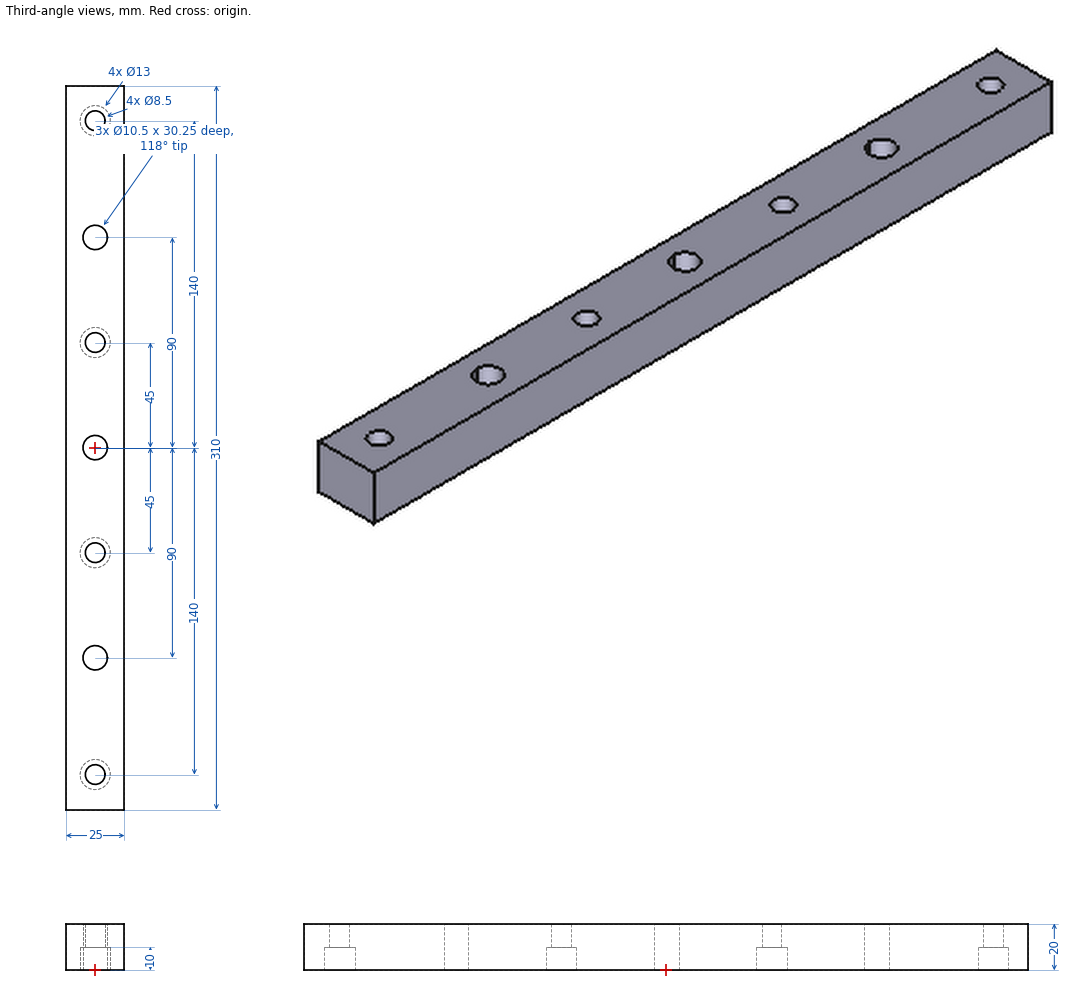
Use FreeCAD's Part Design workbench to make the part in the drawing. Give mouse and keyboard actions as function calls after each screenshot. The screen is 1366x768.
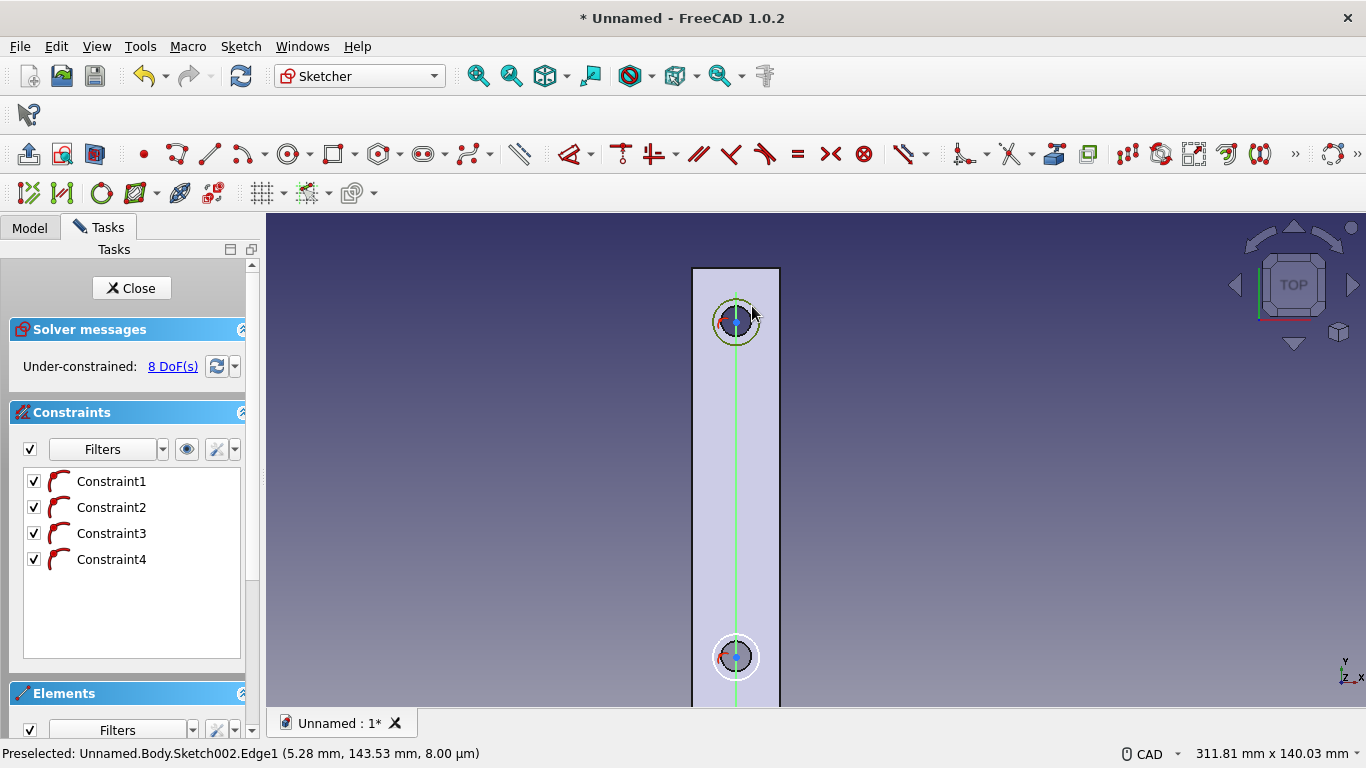
click(752, 641)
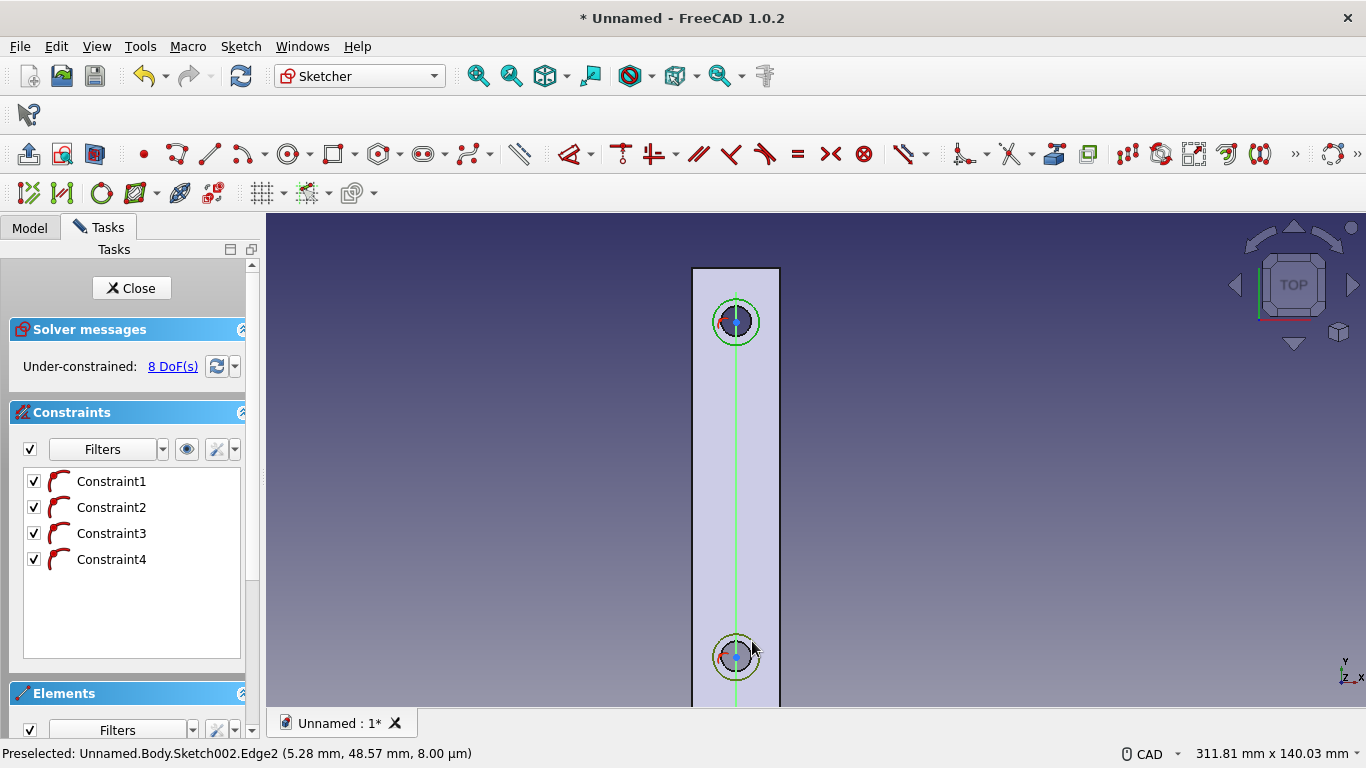
scroll(752, 307, down, 6)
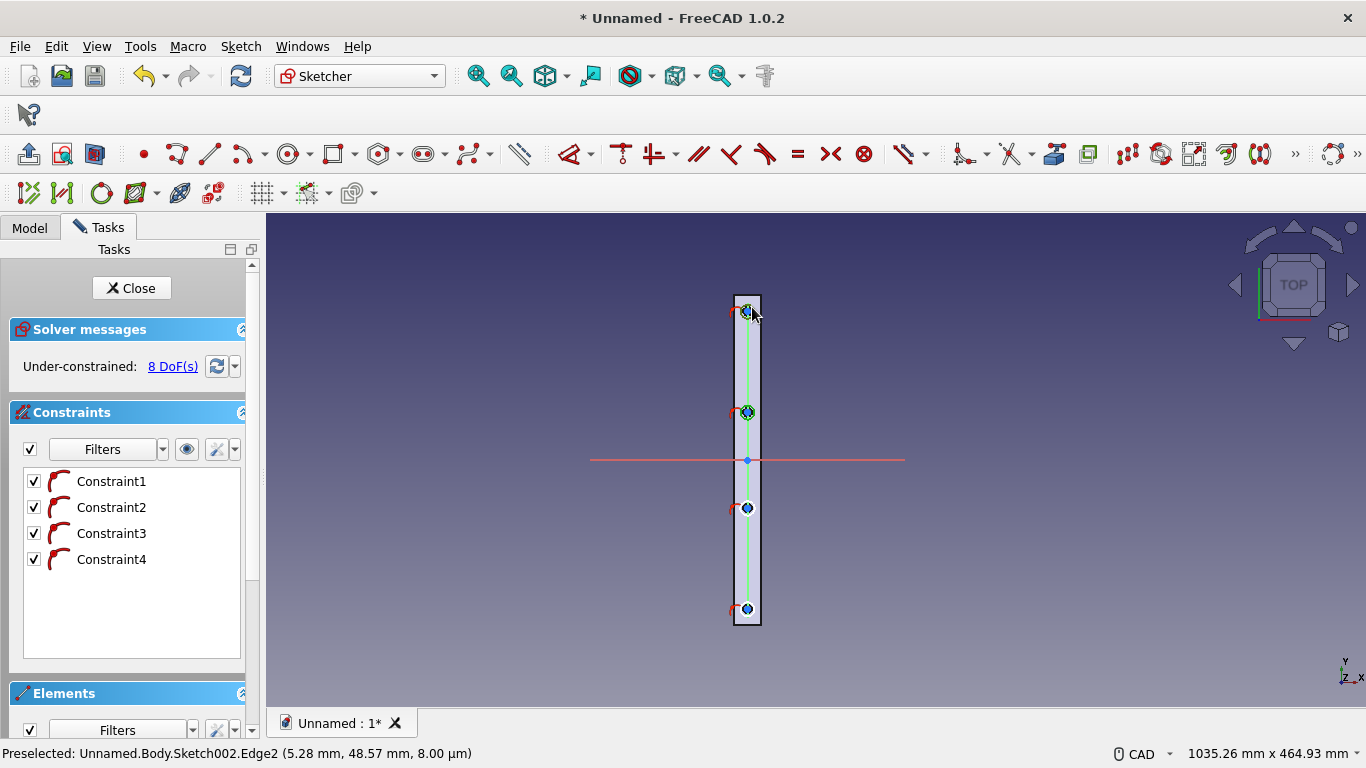
scroll(753, 503, up, 6)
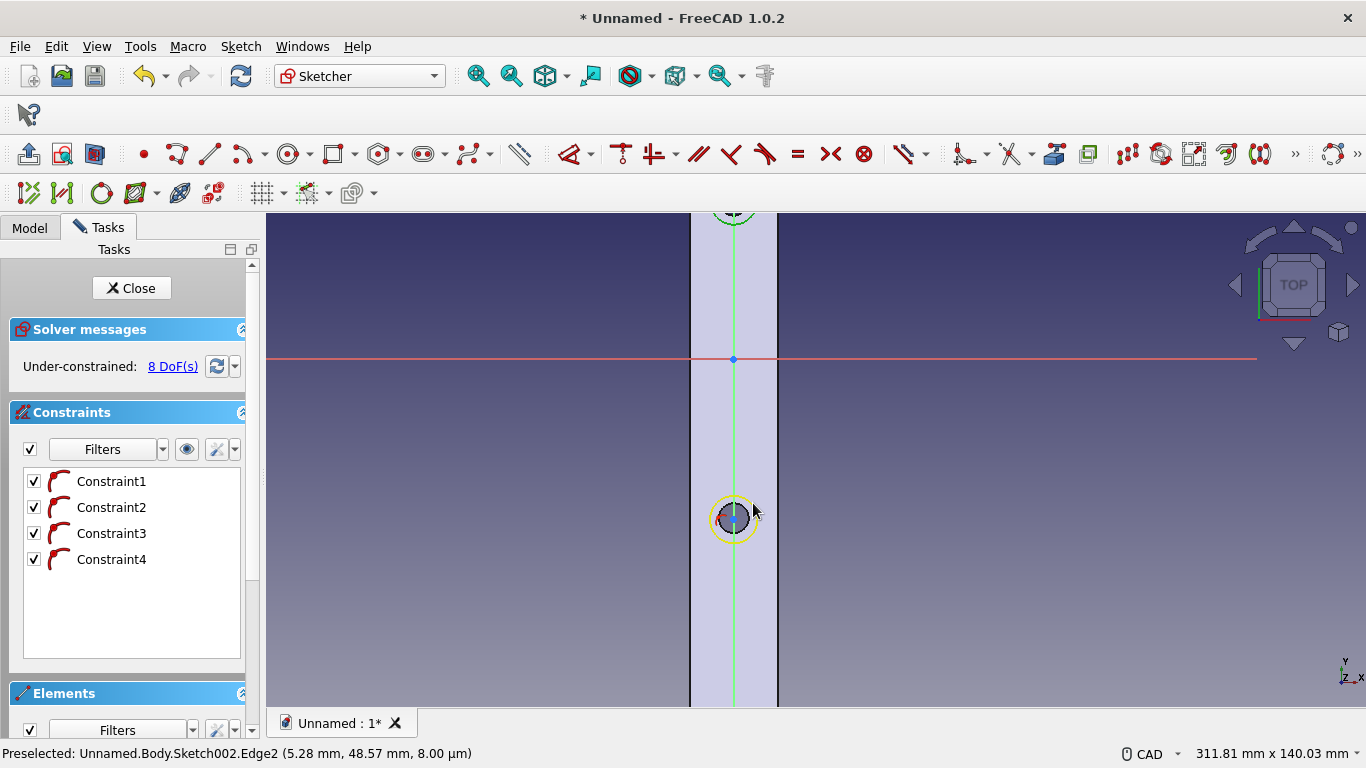
click(751, 503)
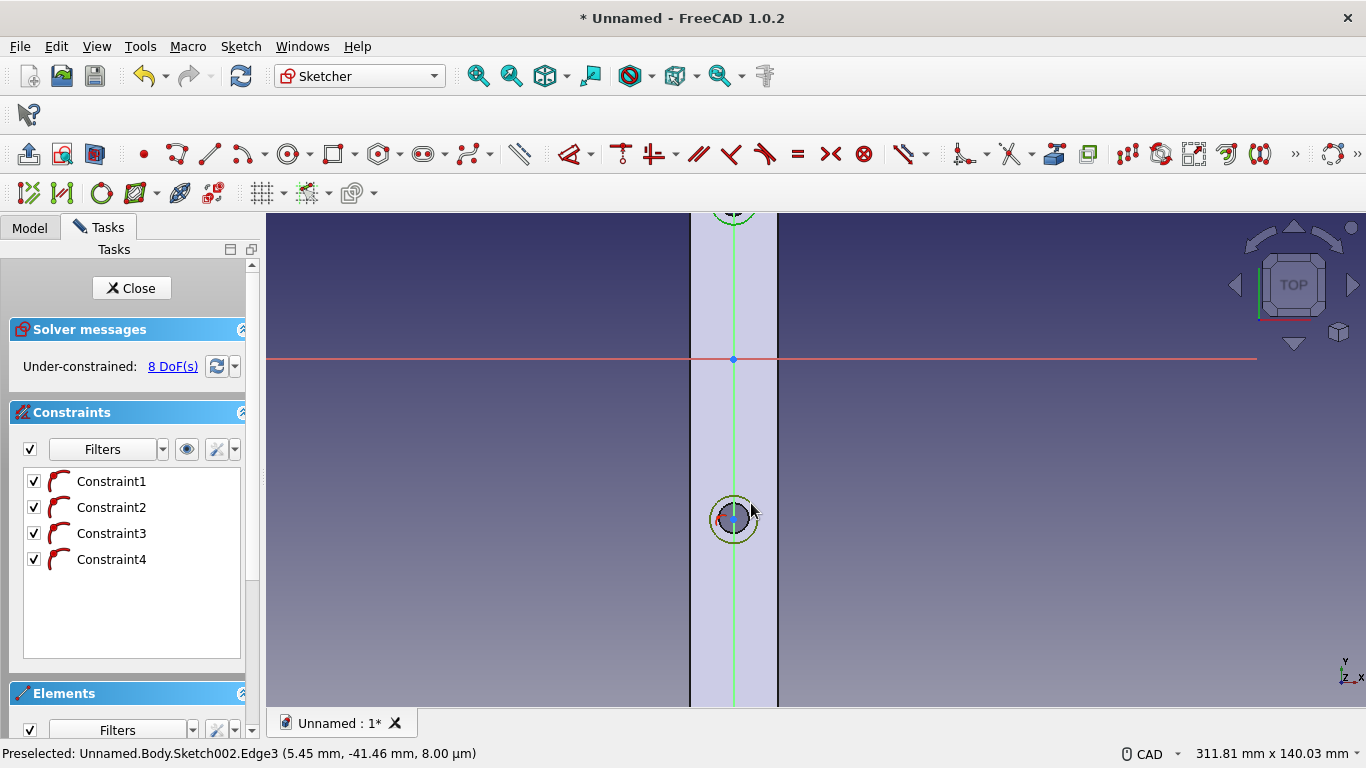
scroll(753, 503, down, 6)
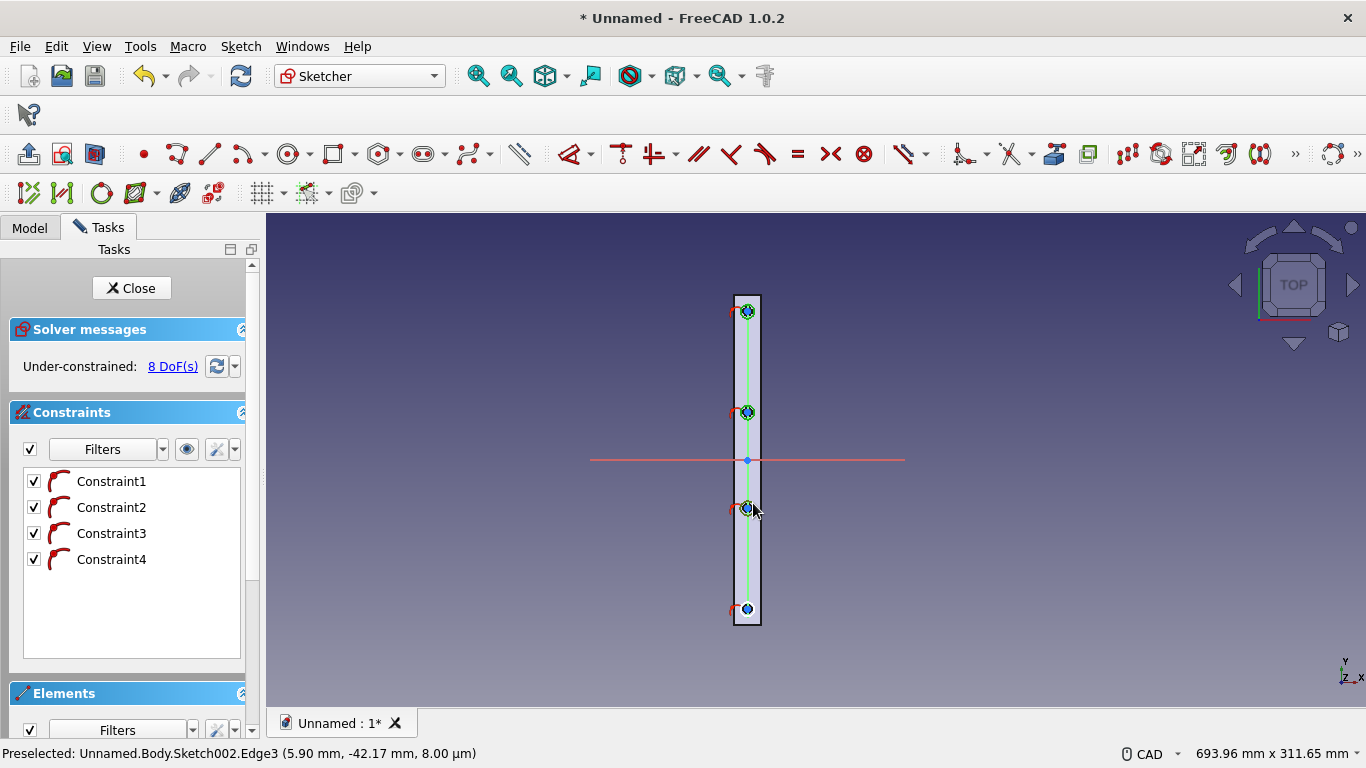
scroll(752, 604, up, 6)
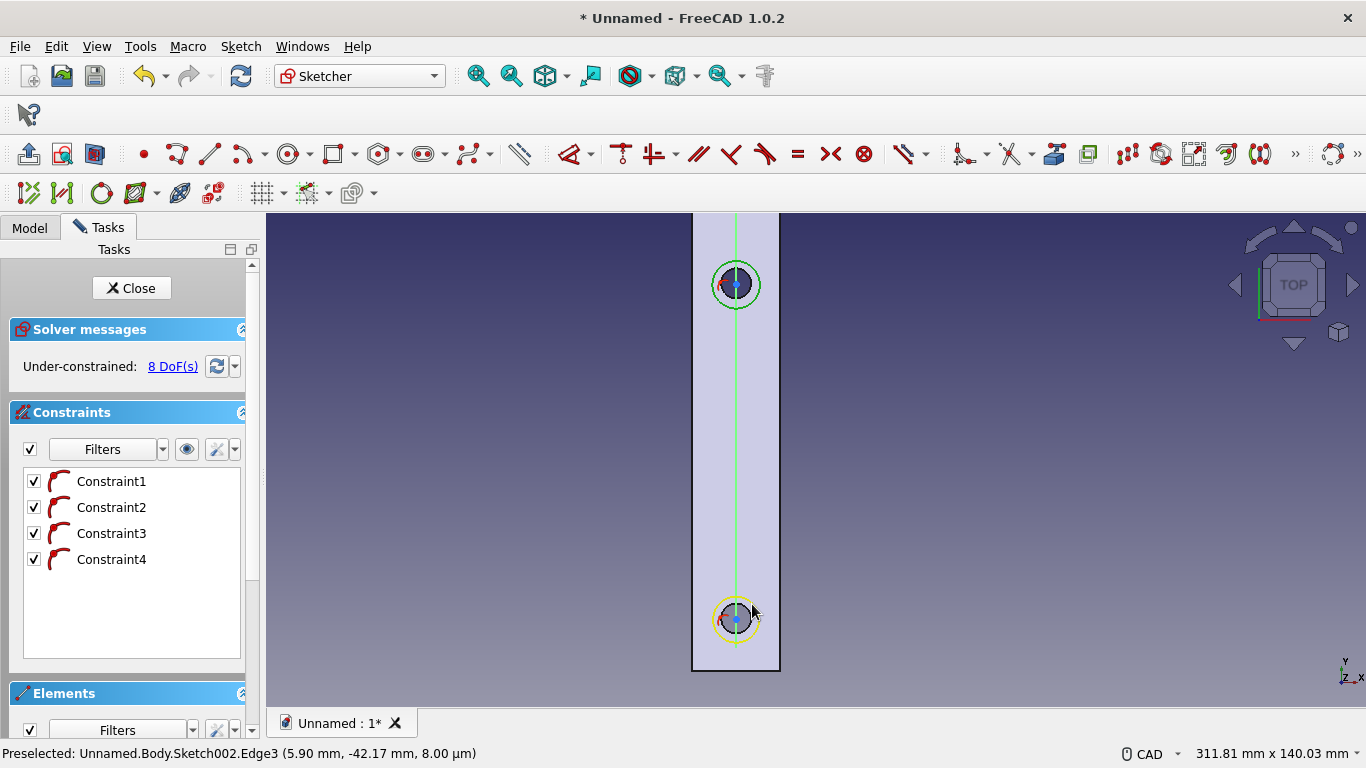
click(752, 603)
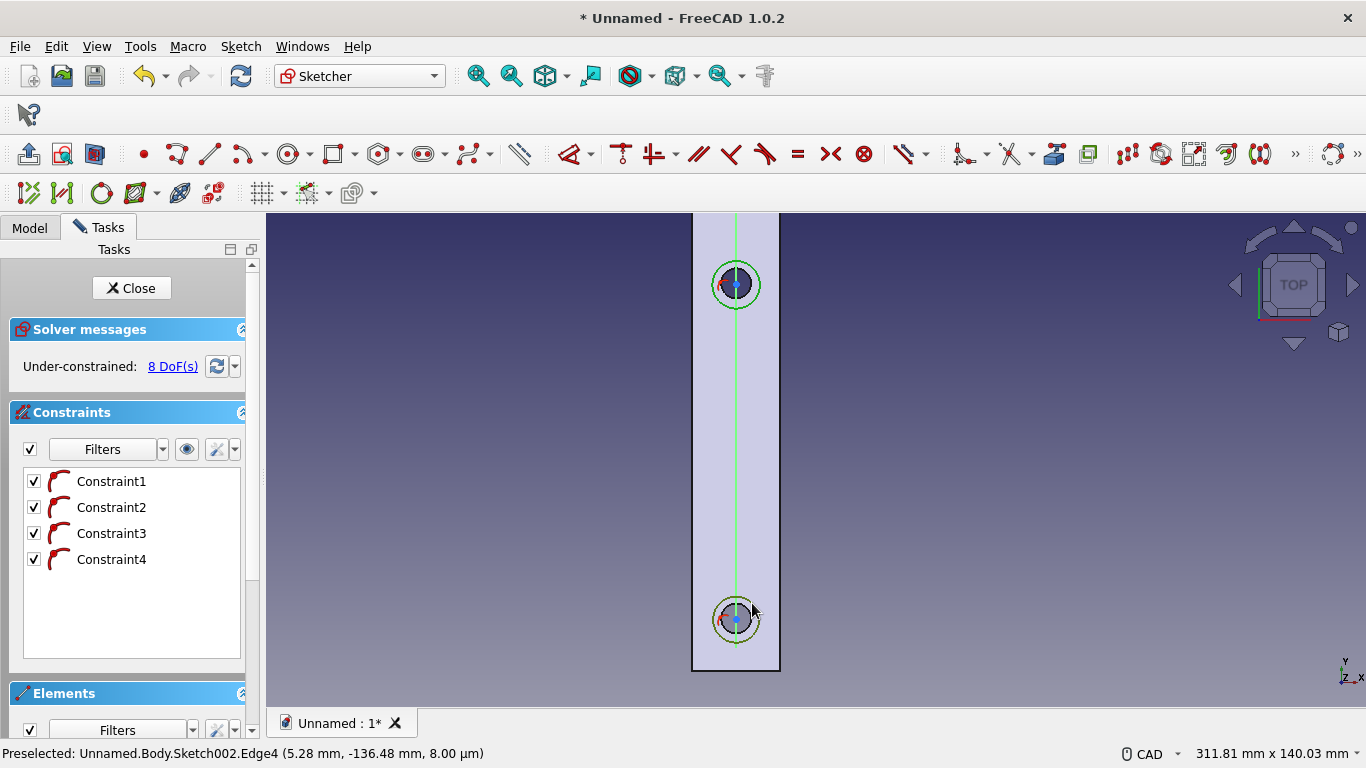
click(798, 154)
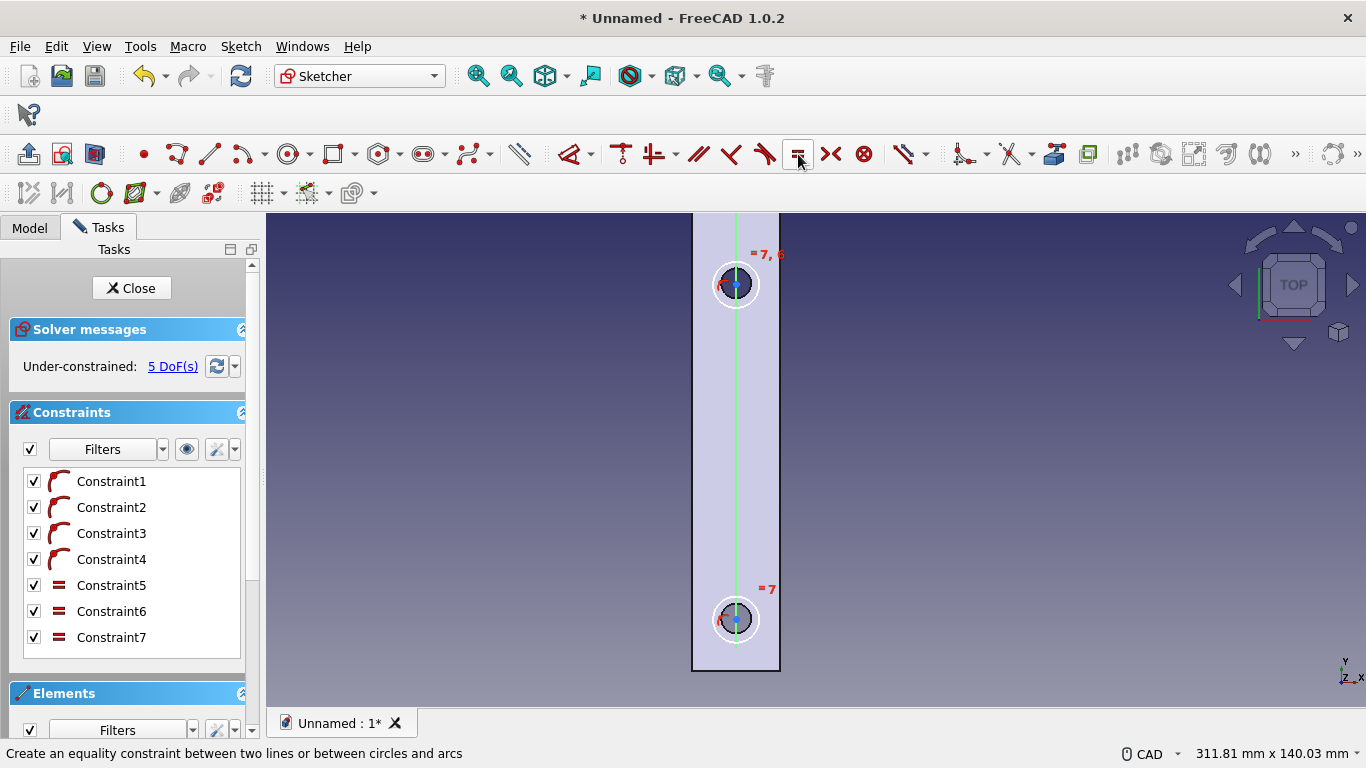
key(d)